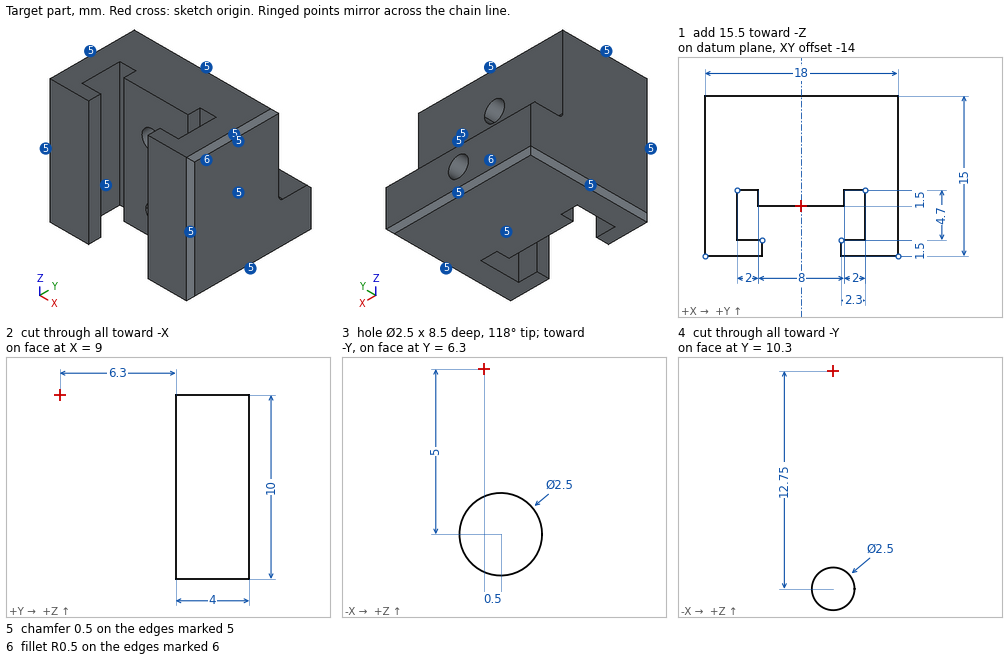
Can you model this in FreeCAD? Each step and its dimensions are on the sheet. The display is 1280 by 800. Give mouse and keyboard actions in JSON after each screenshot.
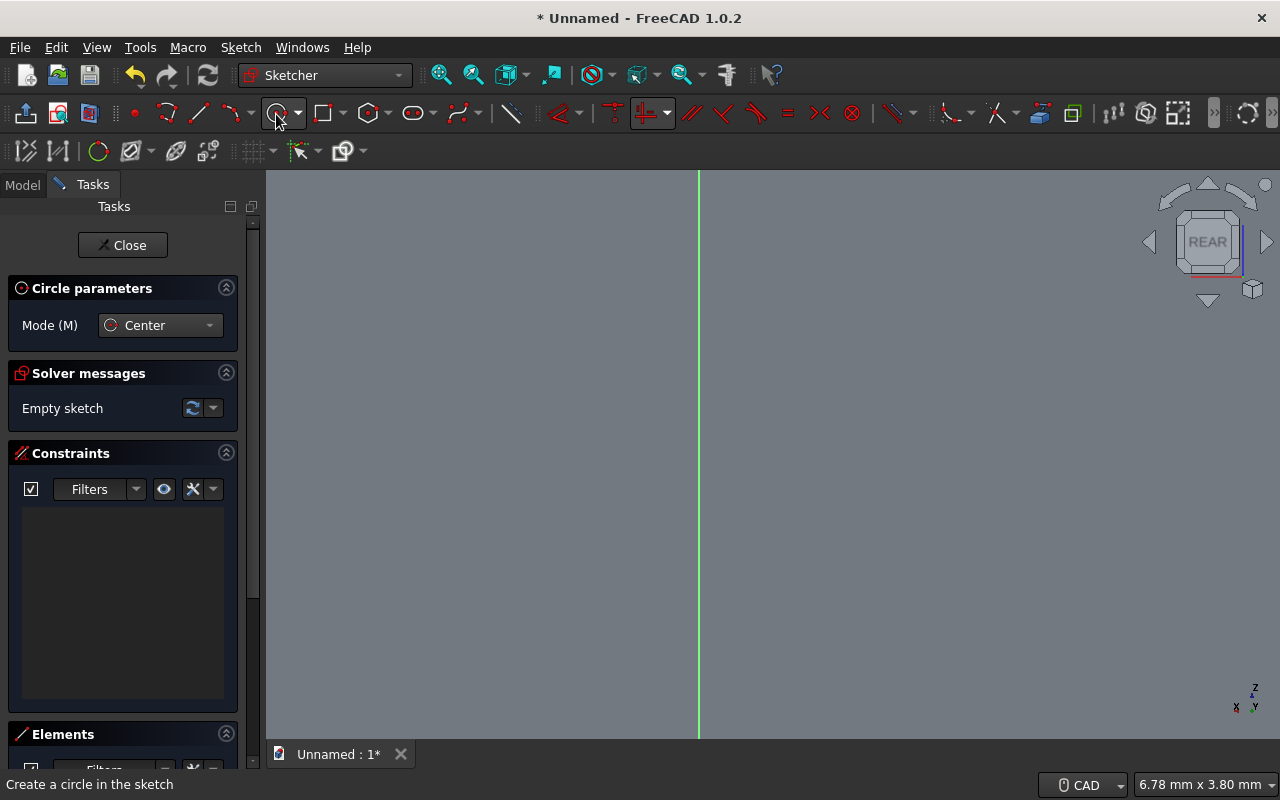
{"action": "left_click", "coordinate": [699, 448]}
{"action": "mouse_move", "coordinate": [832, 315]}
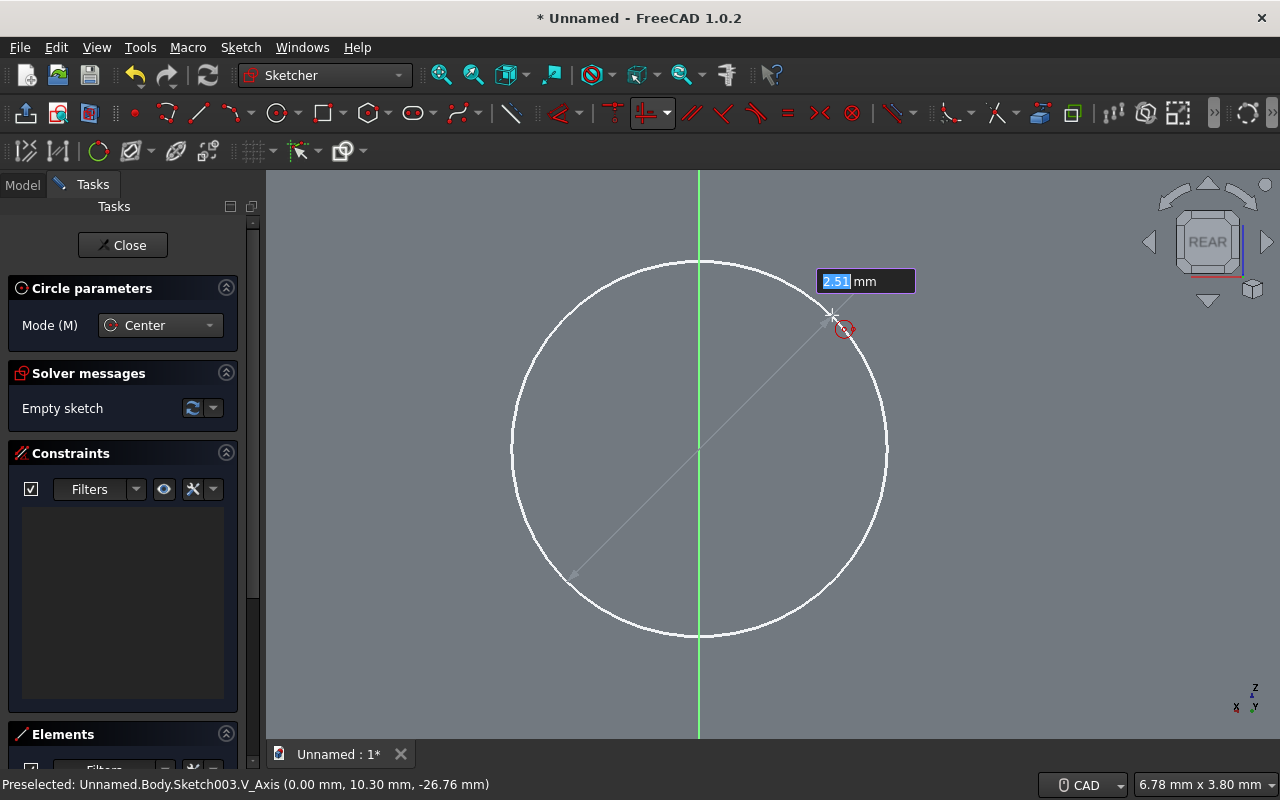
{"action": "type", "text": "2.5"}
{"action": "key", "text": "Return"}
{"action": "key", "text": "Escape"}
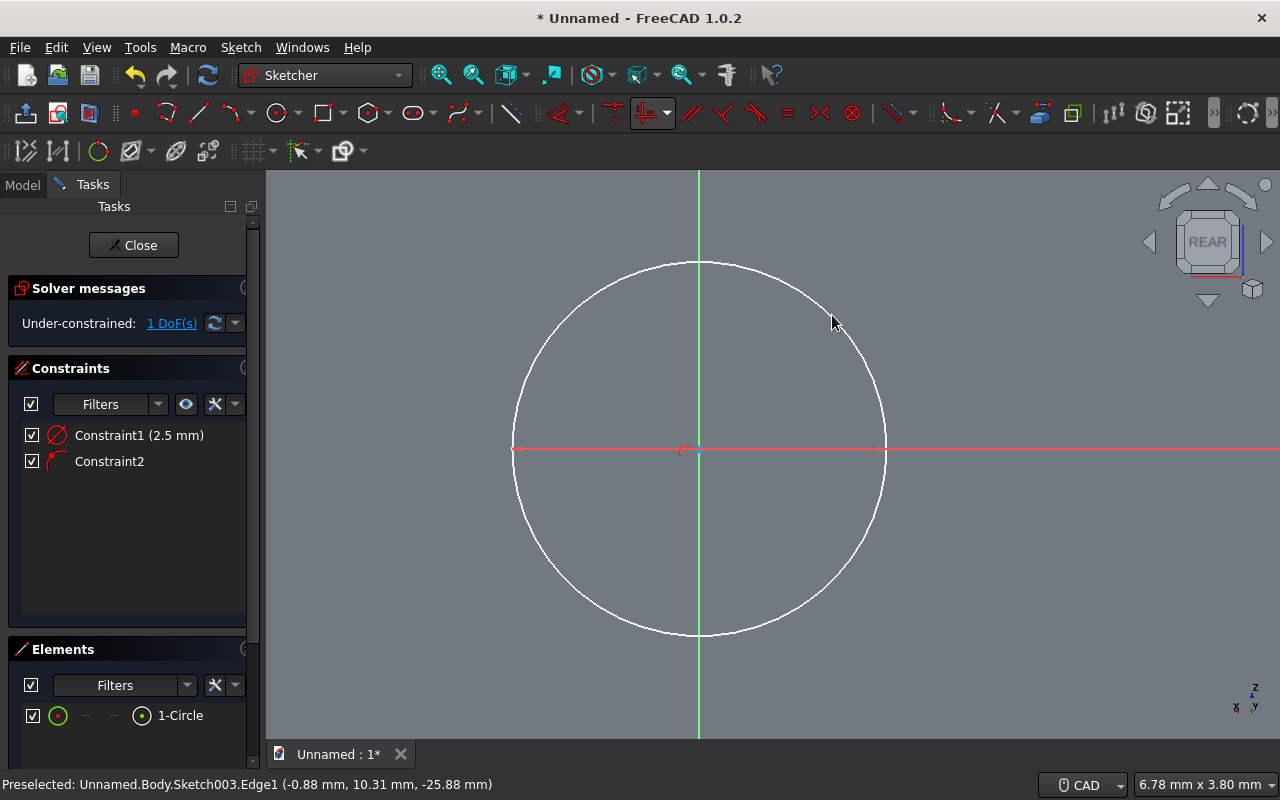
{"action": "left_click", "coordinate": [558, 114]}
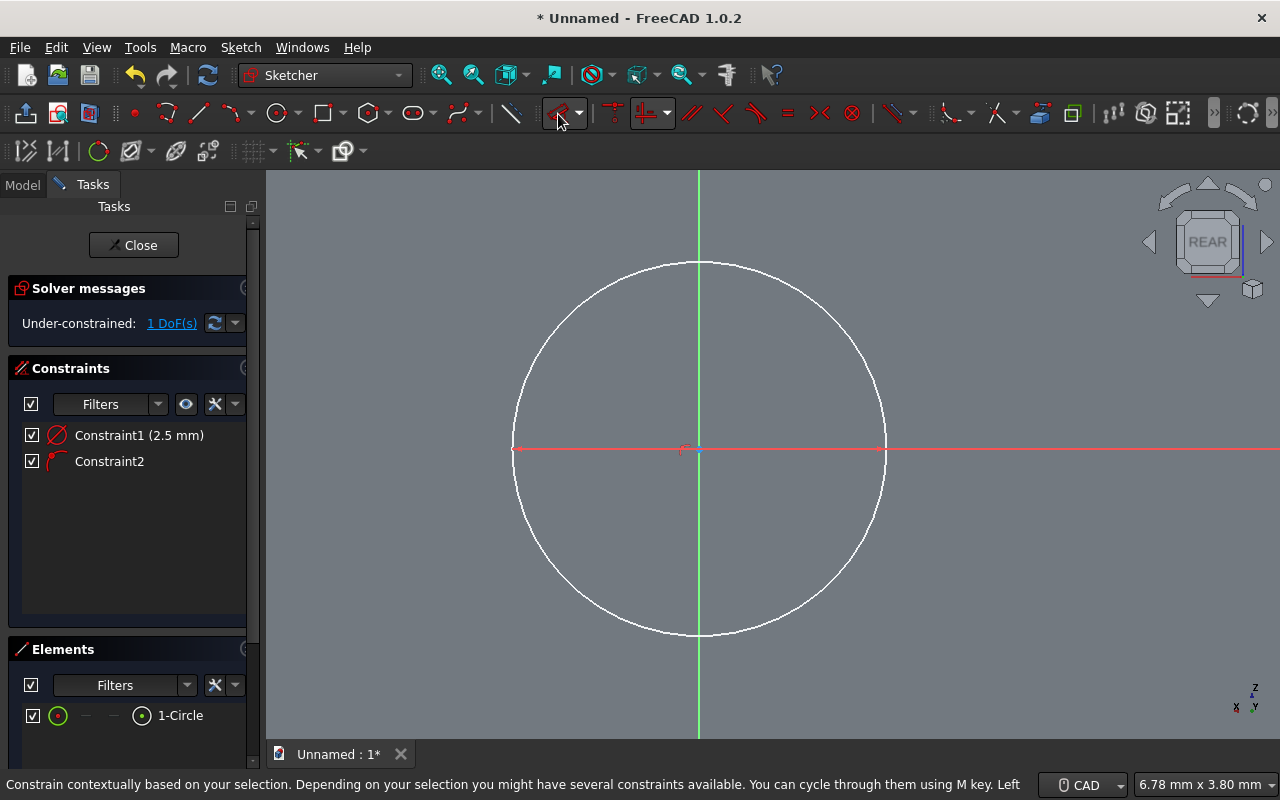
{"action": "left_click", "coordinate": [699, 449]}
{"action": "left_click", "coordinate": [733, 324]}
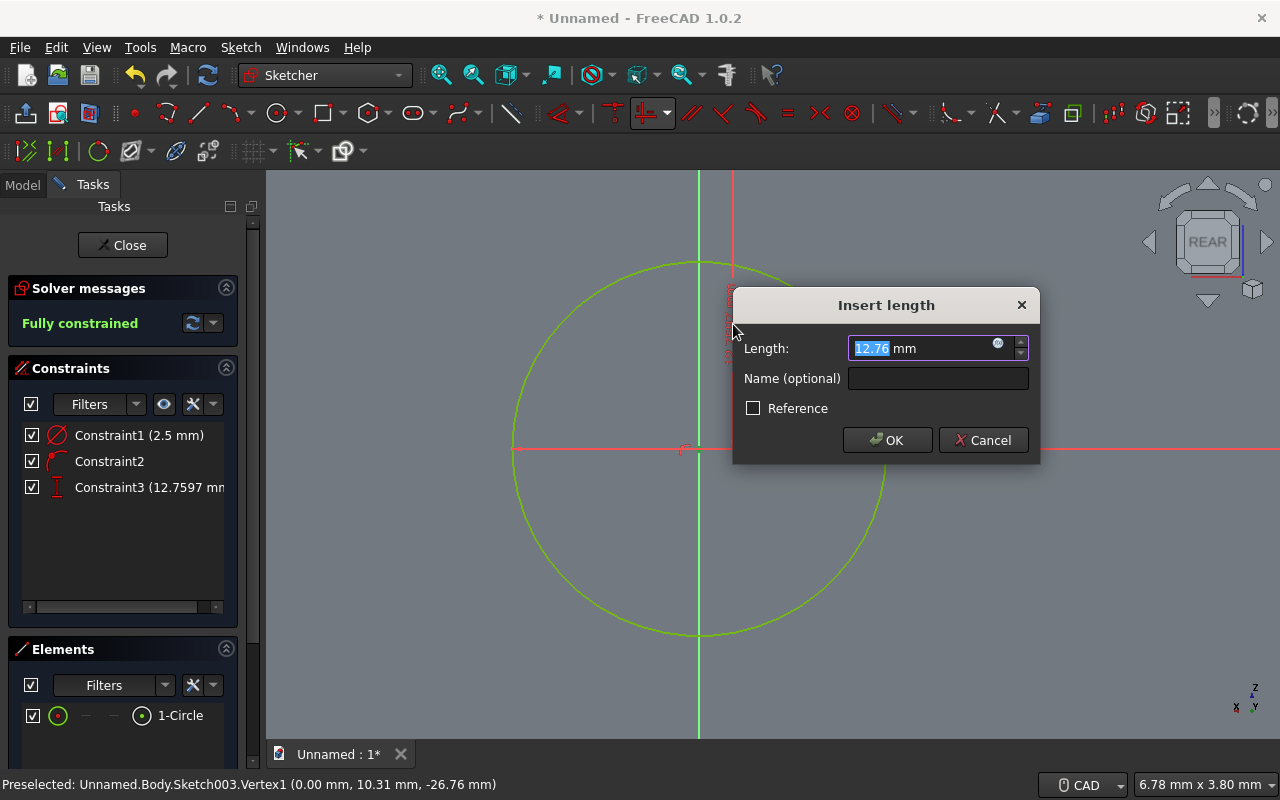
{"action": "type", "text": "12.75"}
{"action": "key", "text": "Return"}
{"action": "key", "text": "Escape"}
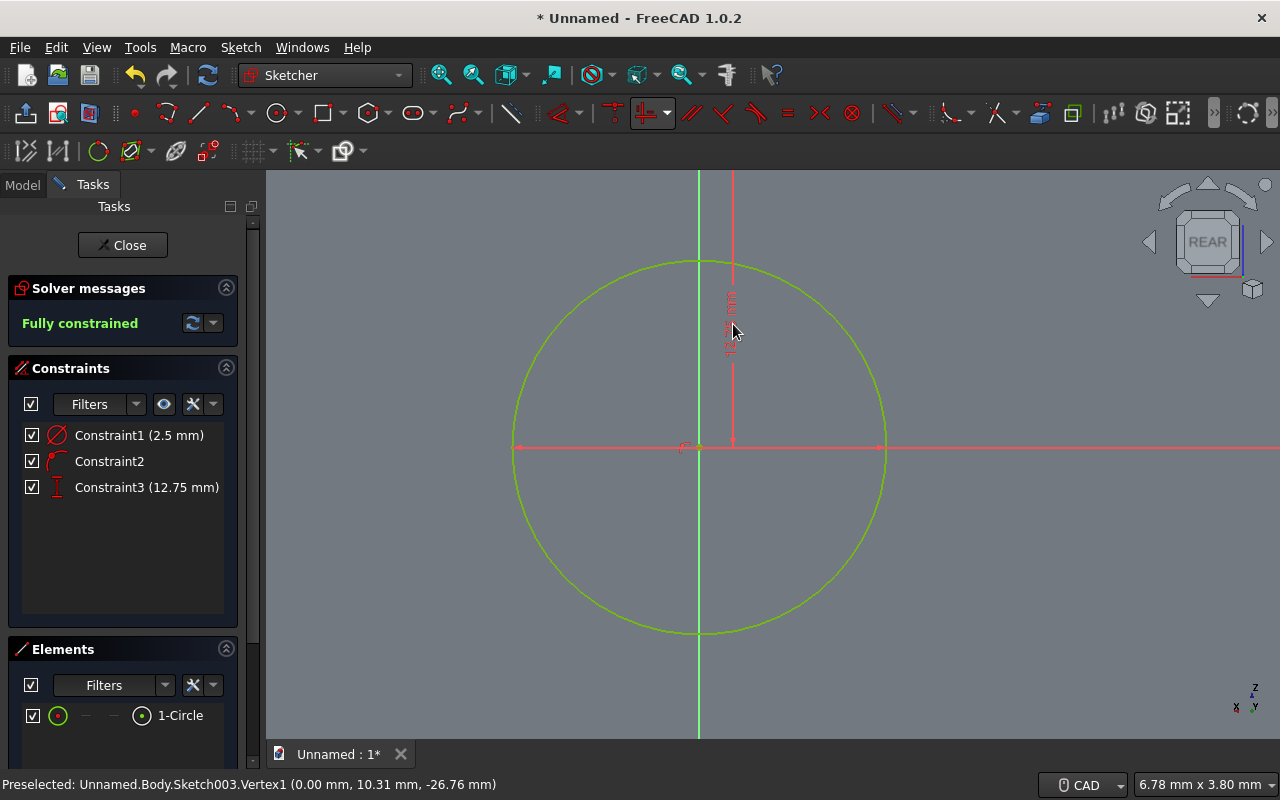
{"action": "left_click", "coordinate": [123, 245]}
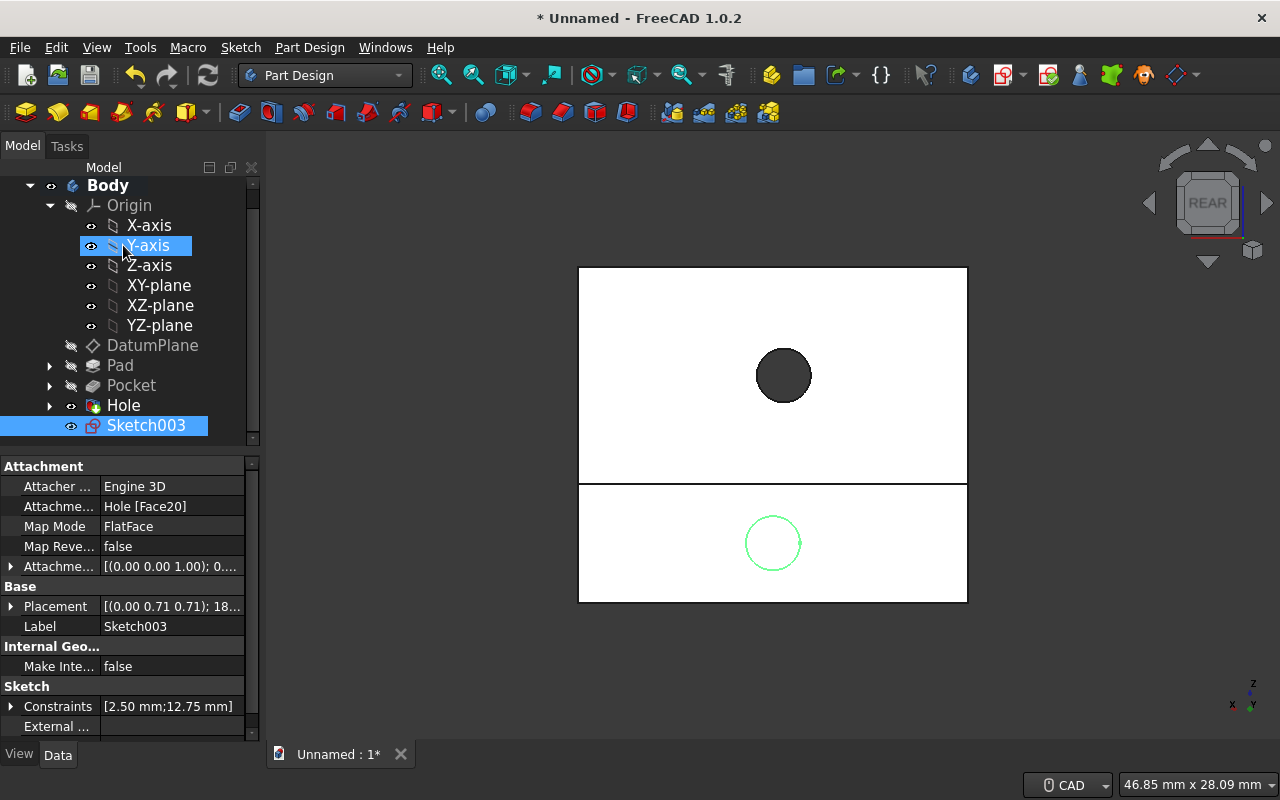
{"action": "left_click", "coordinate": [240, 112]}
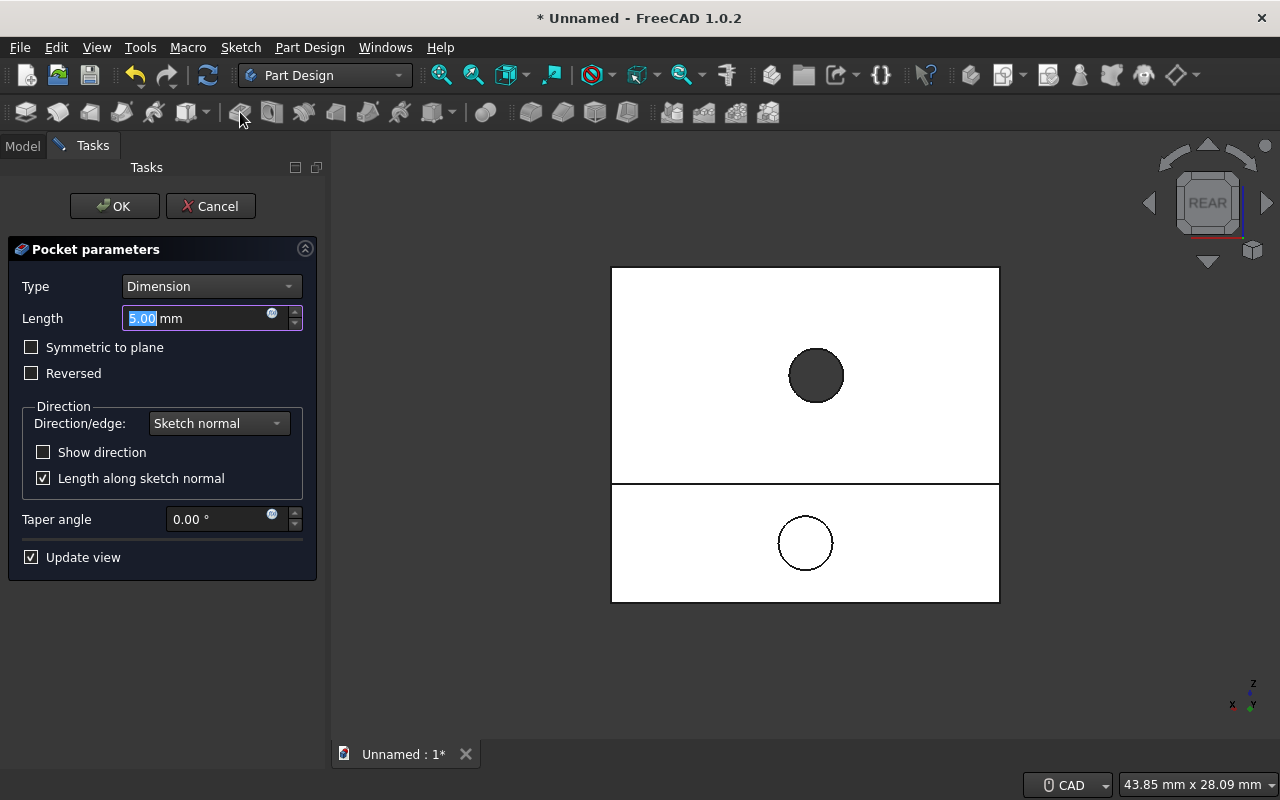
{"action": "left_click", "coordinate": [212, 286]}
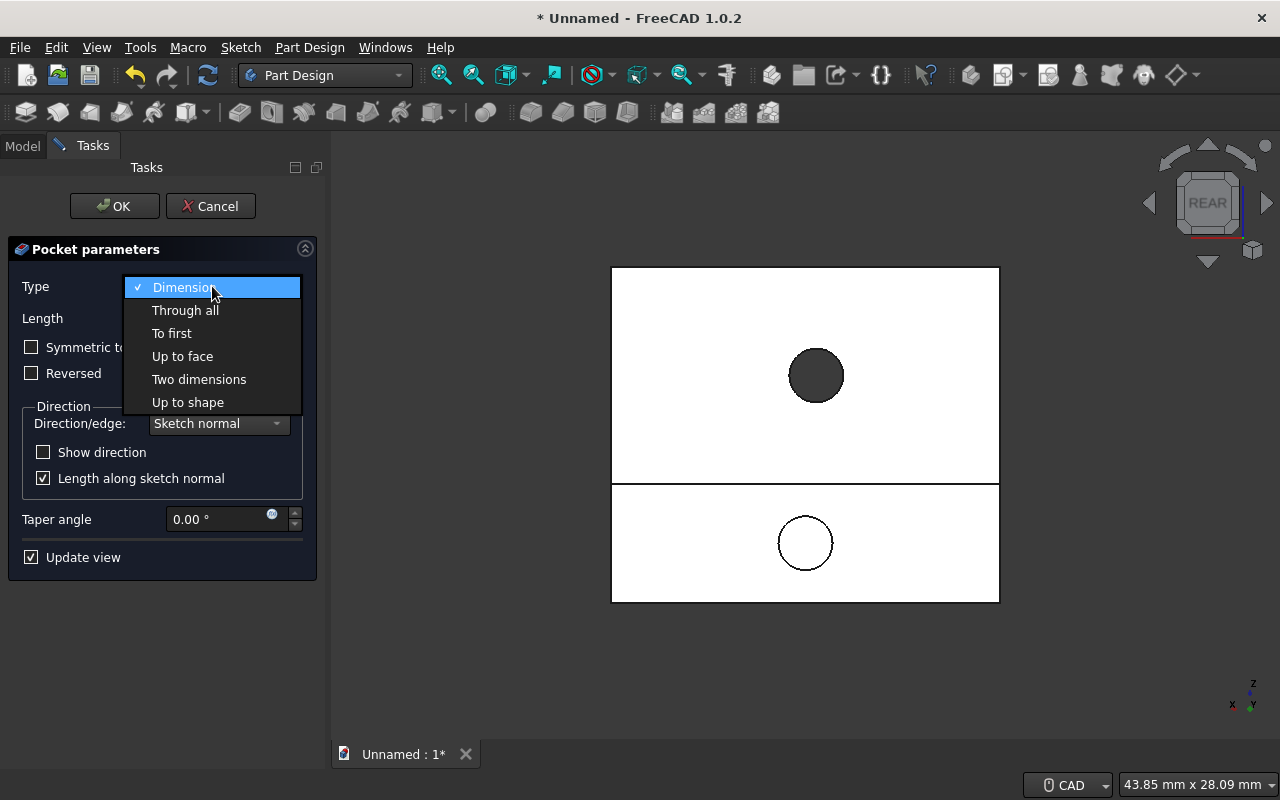
{"action": "left_click", "coordinate": [212, 310]}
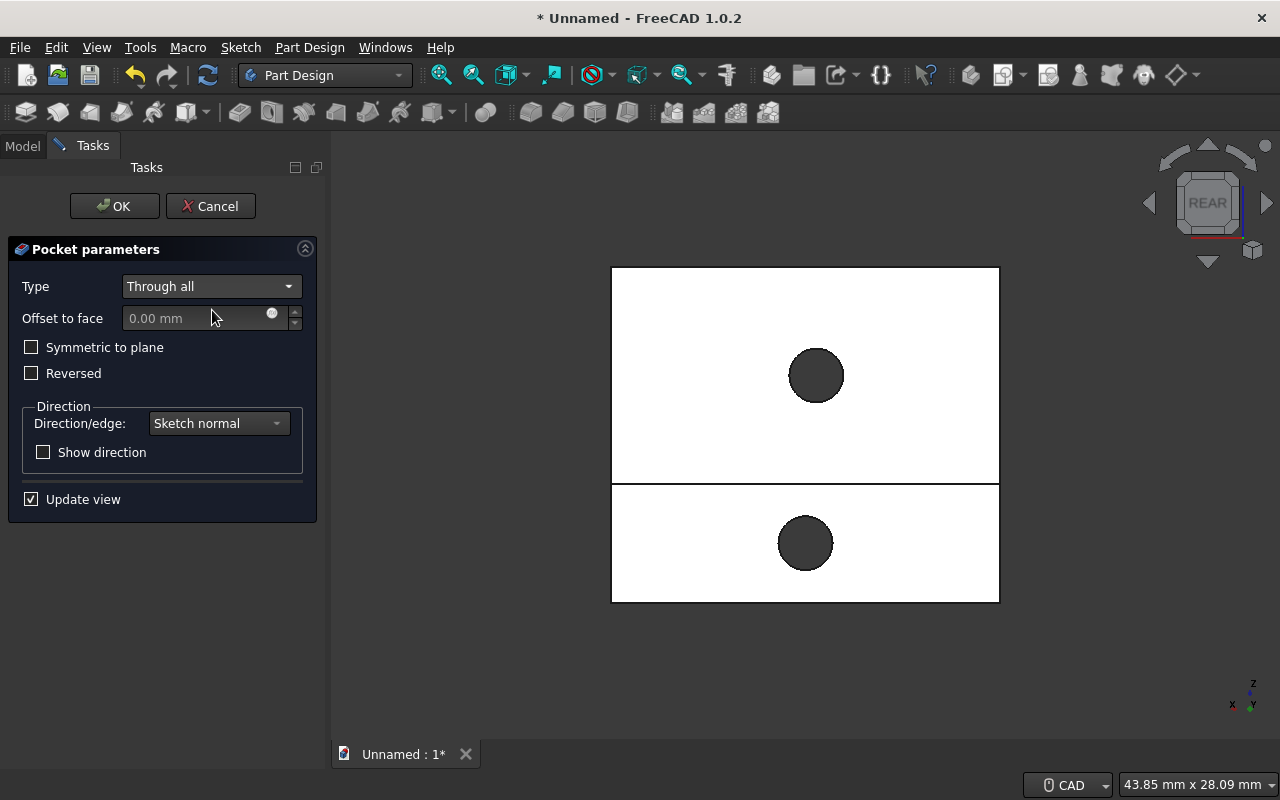
{"action": "left_click", "coordinate": [115, 206]}